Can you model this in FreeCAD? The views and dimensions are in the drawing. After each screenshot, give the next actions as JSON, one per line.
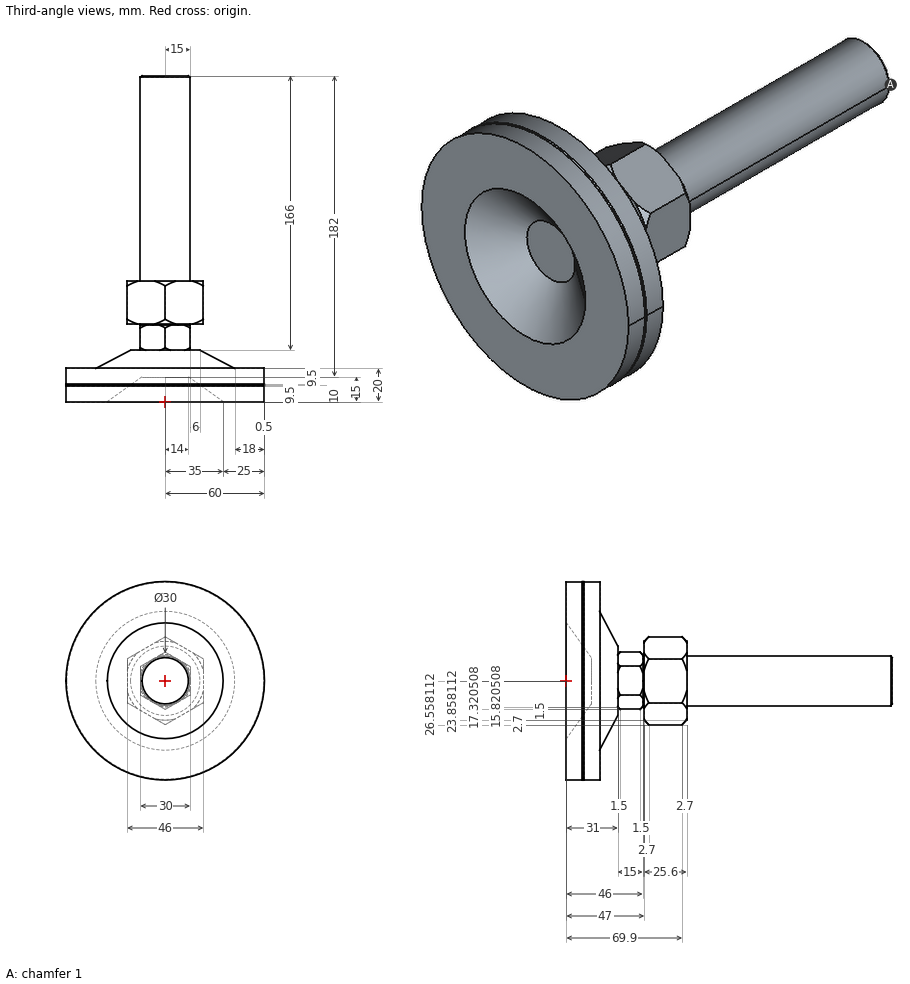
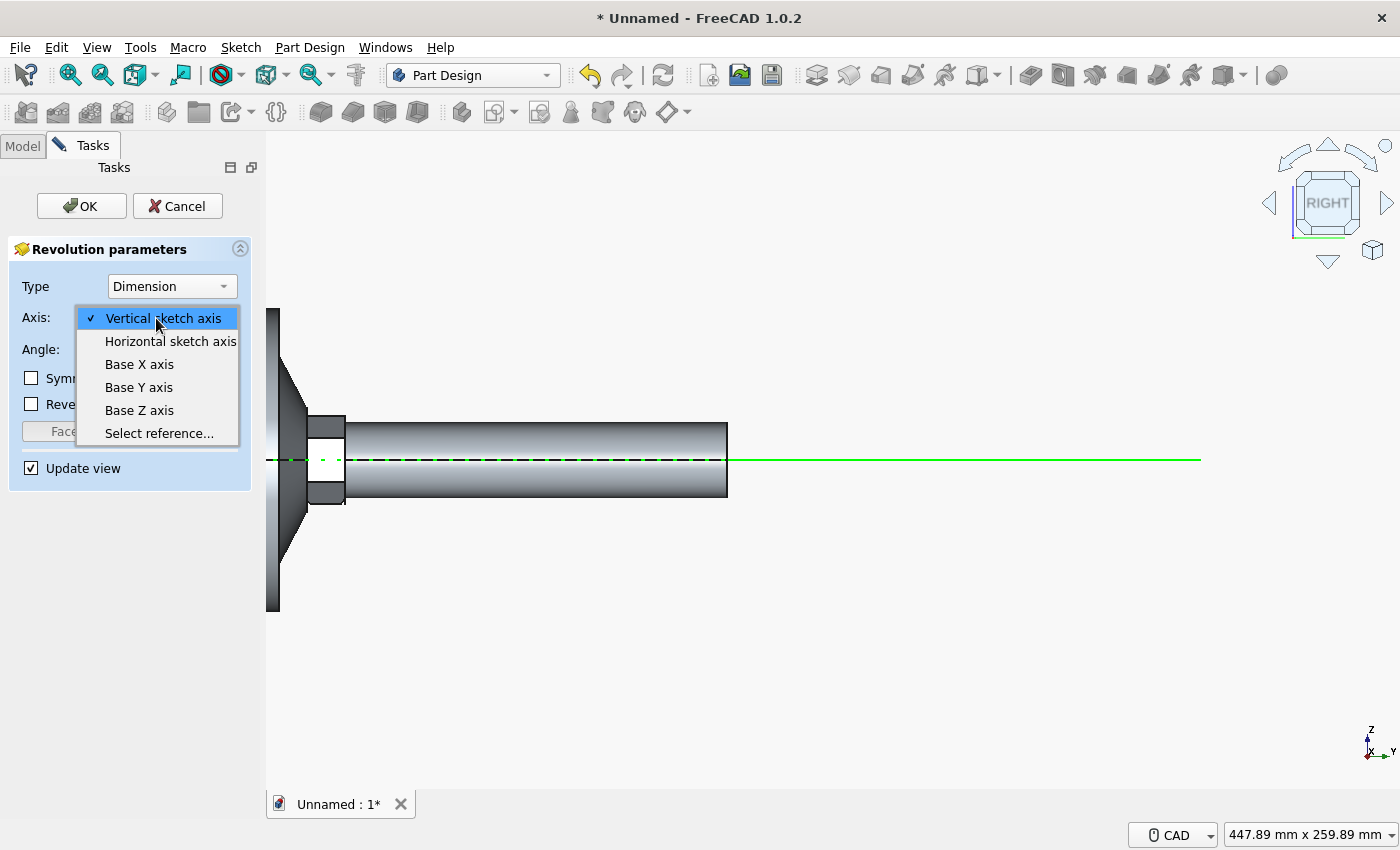
{"action": "left_click", "coordinate": [156, 342]}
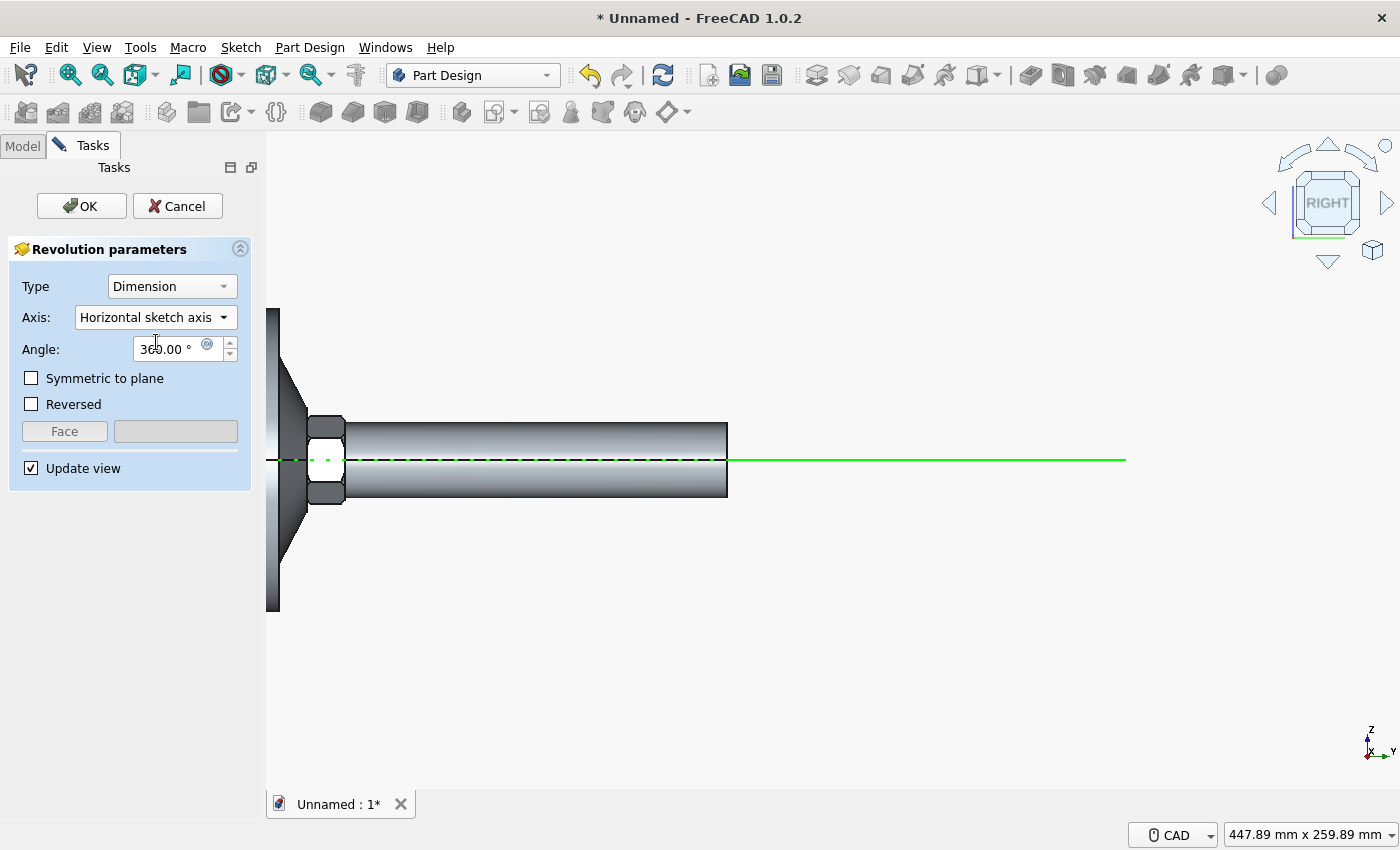
{"action": "left_click", "coordinate": [82, 206]}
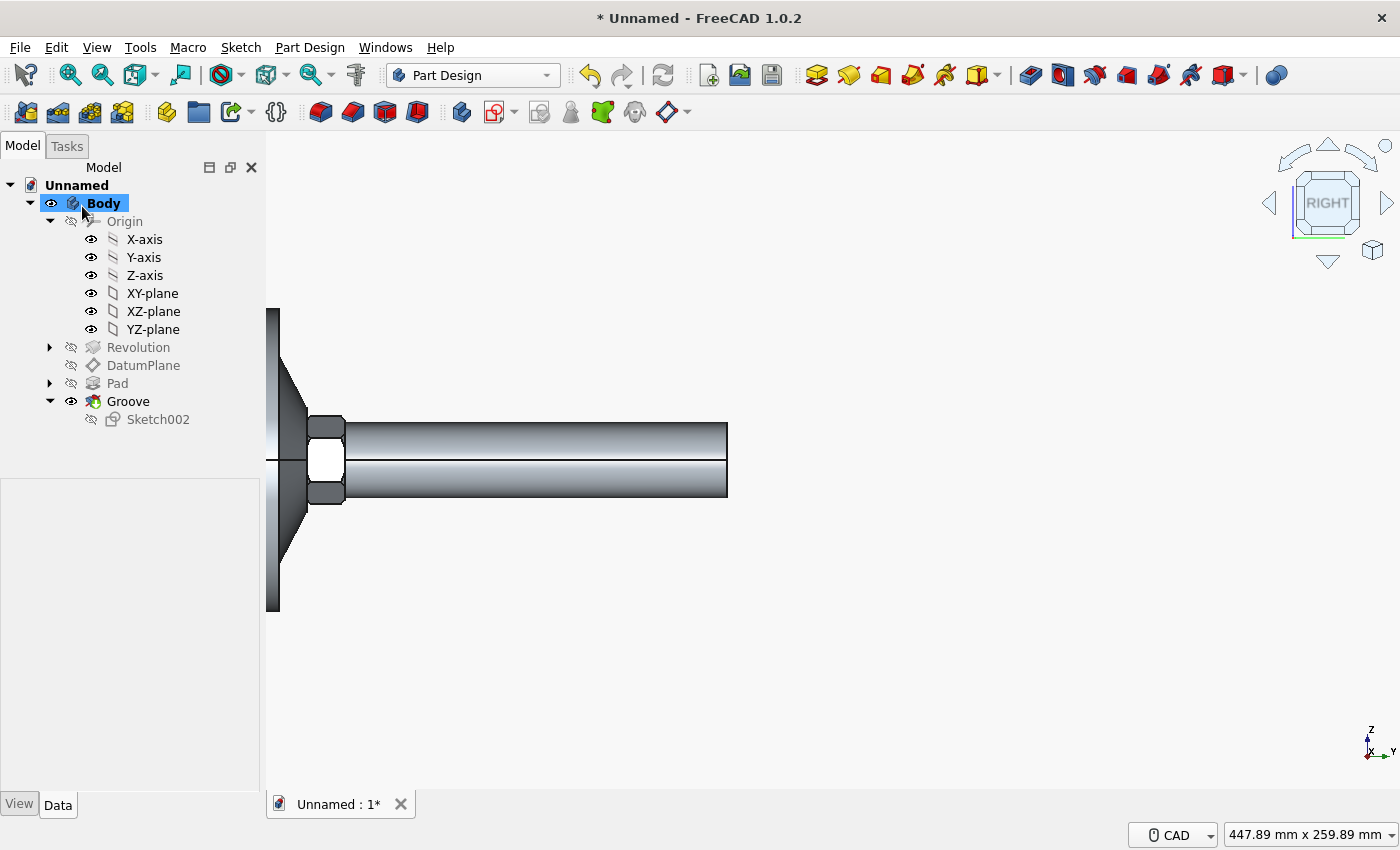
{"action": "left_click", "coordinate": [72, 76]}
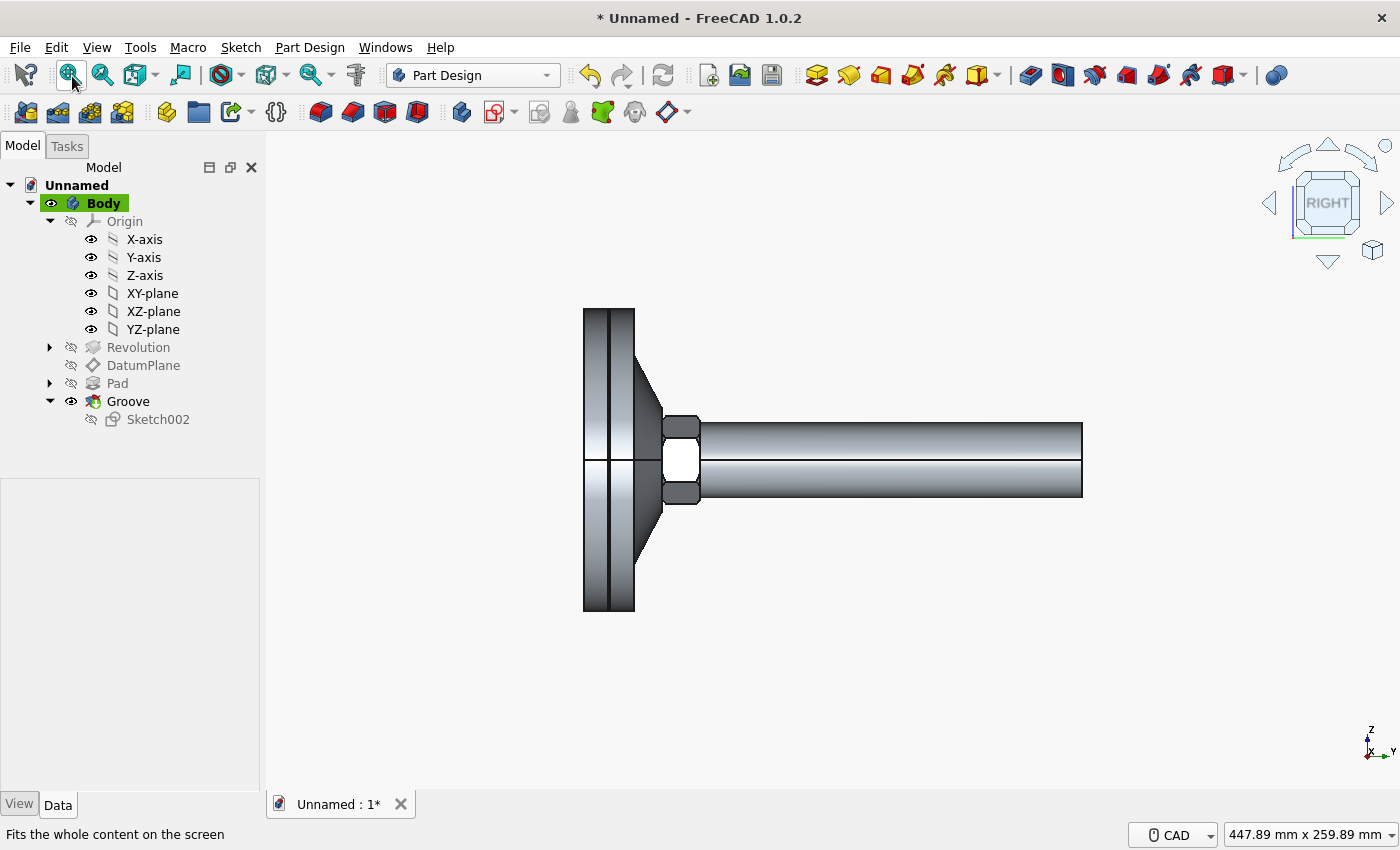
{"action": "left_click", "coordinate": [136, 311]}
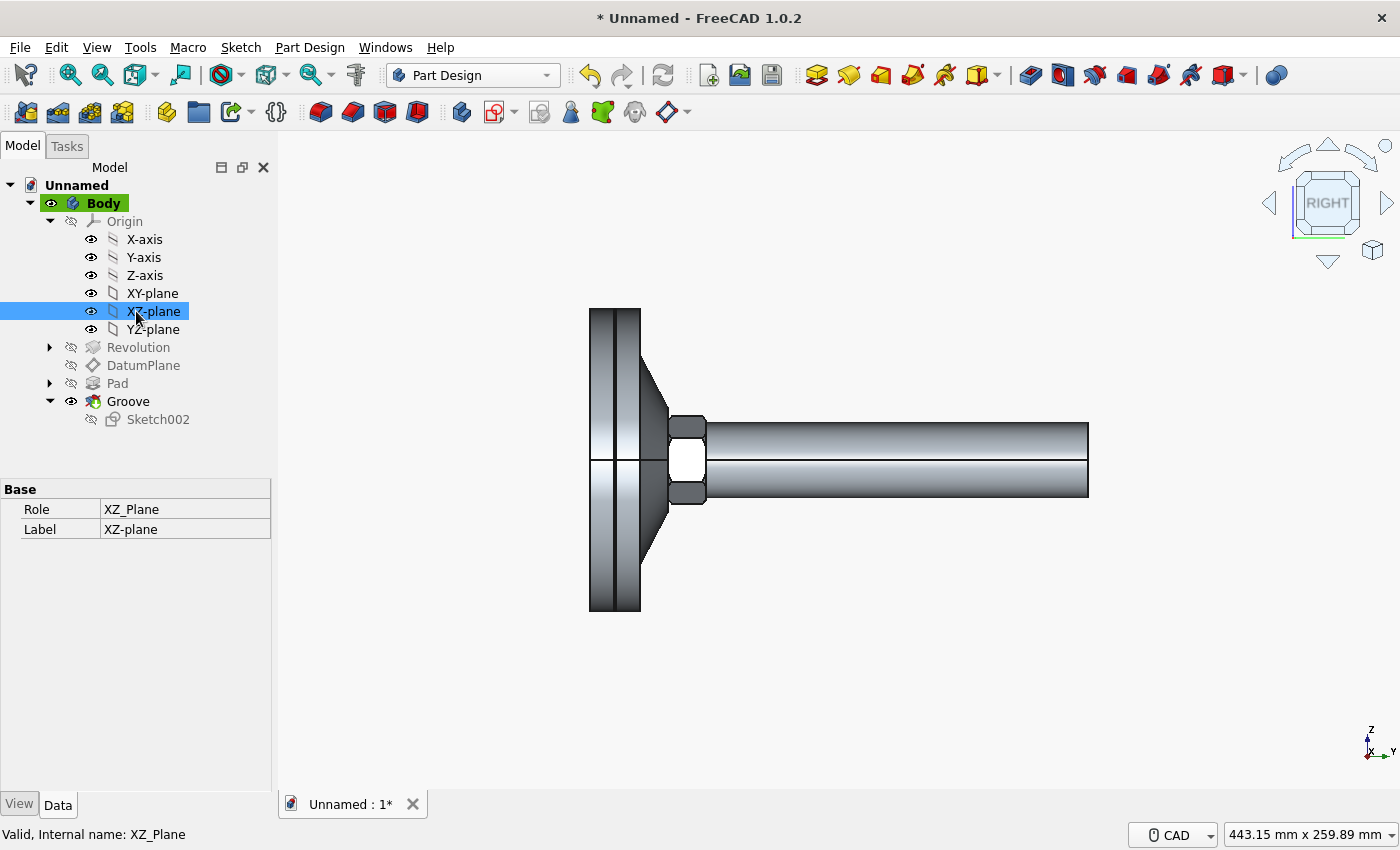
{"action": "left_click", "coordinate": [668, 112]}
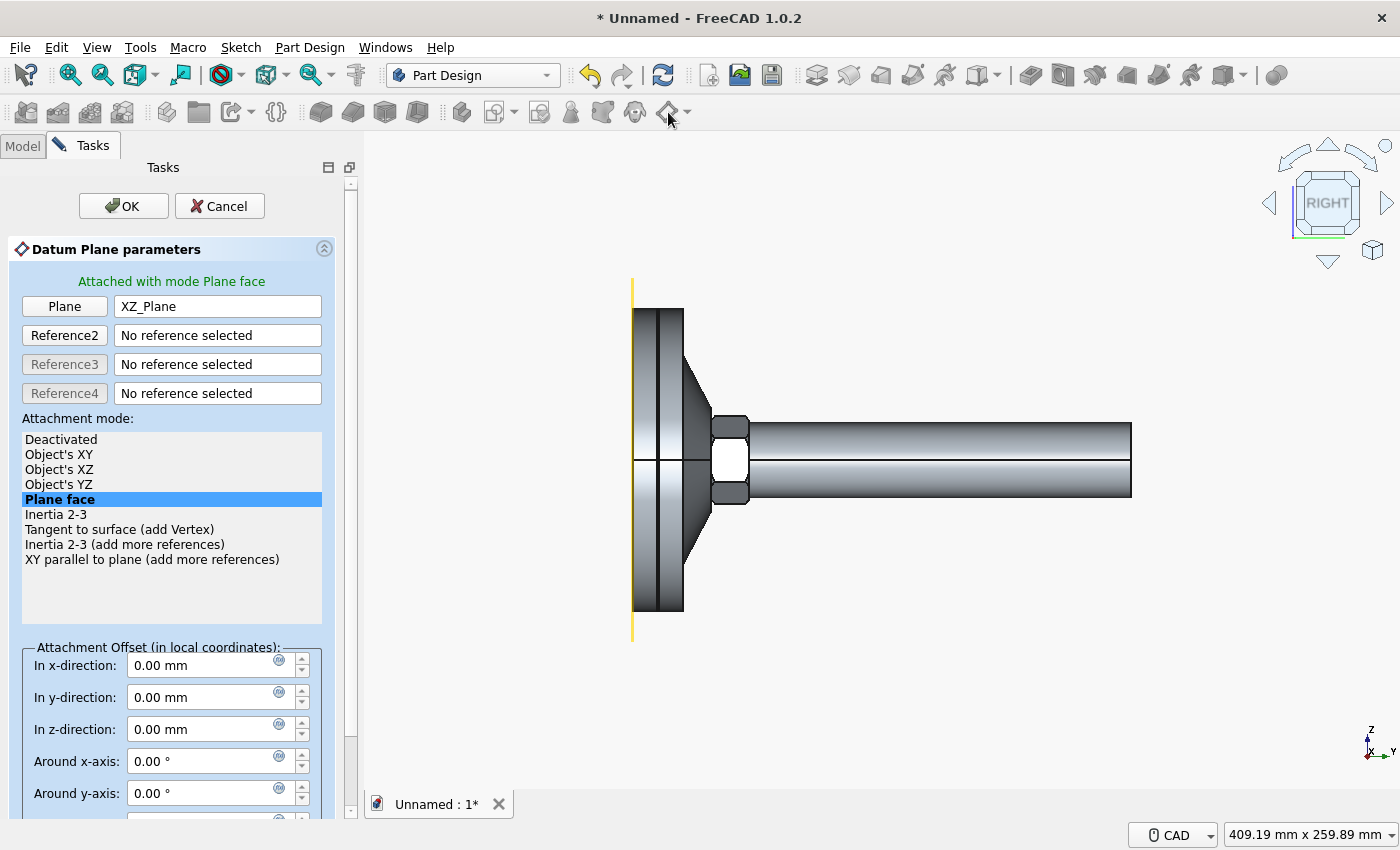
{"action": "triple_click", "coordinate": [210, 729]}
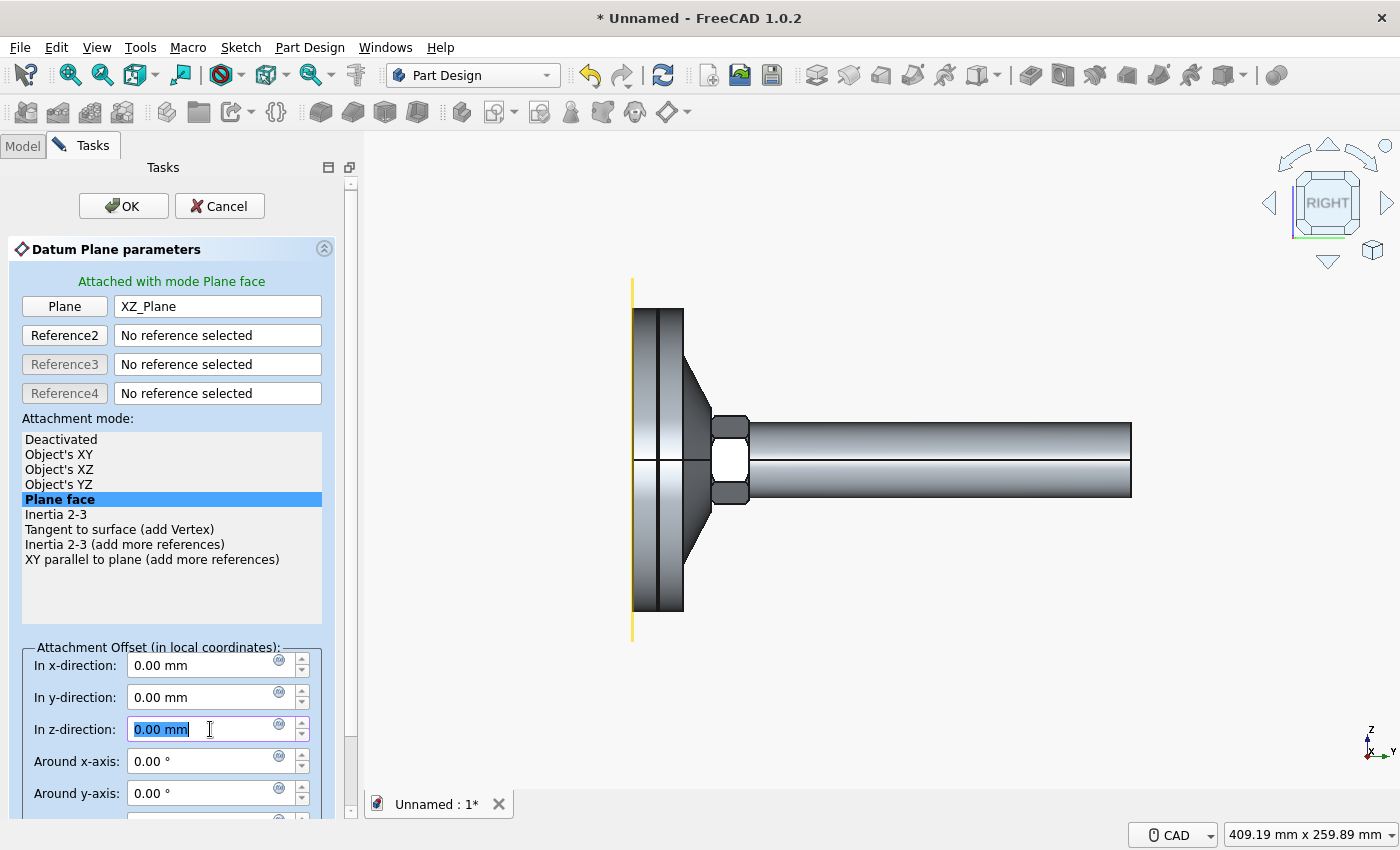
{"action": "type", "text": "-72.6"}
{"action": "key", "text": "Tab"}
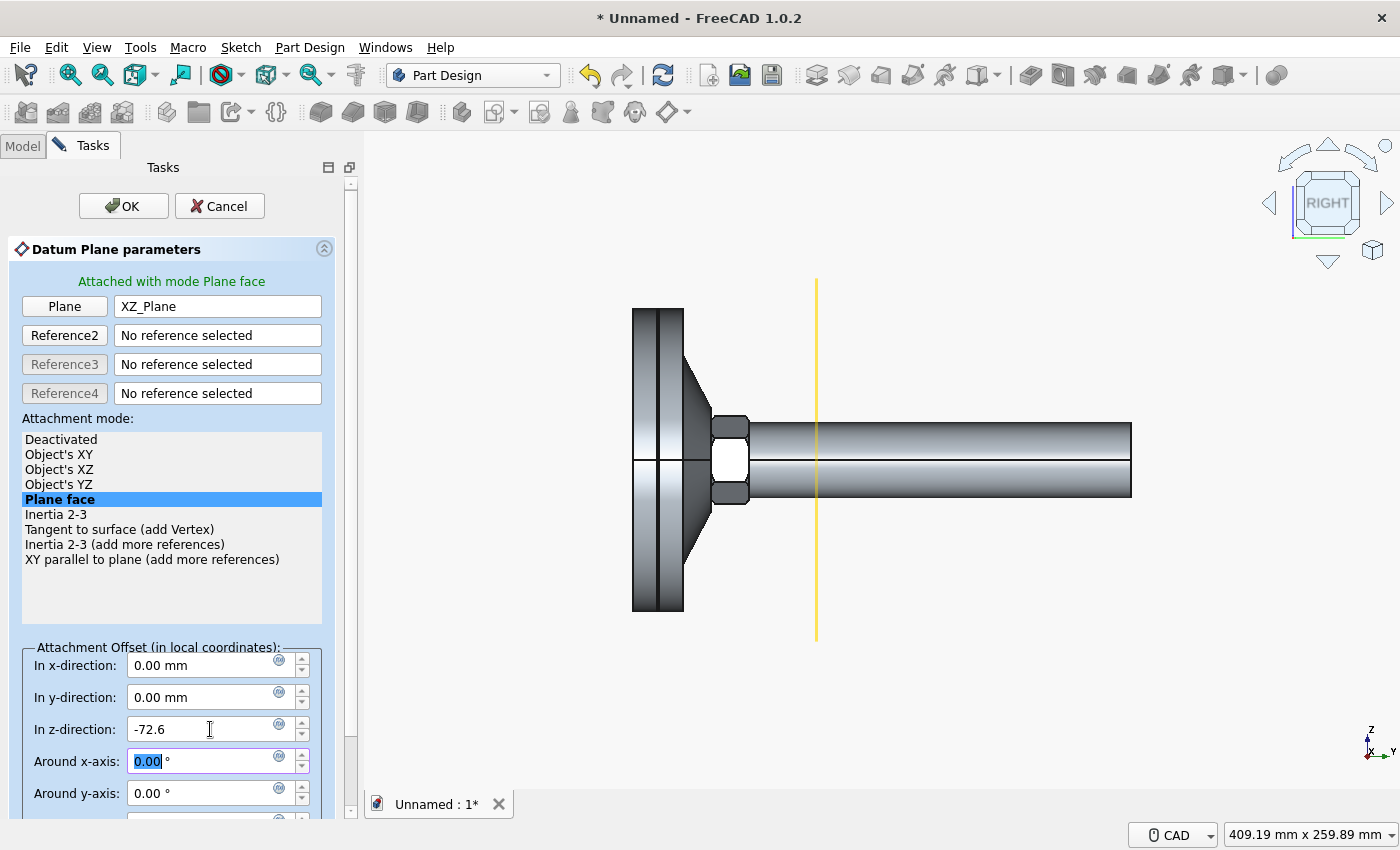
{"action": "left_click", "coordinate": [124, 206]}